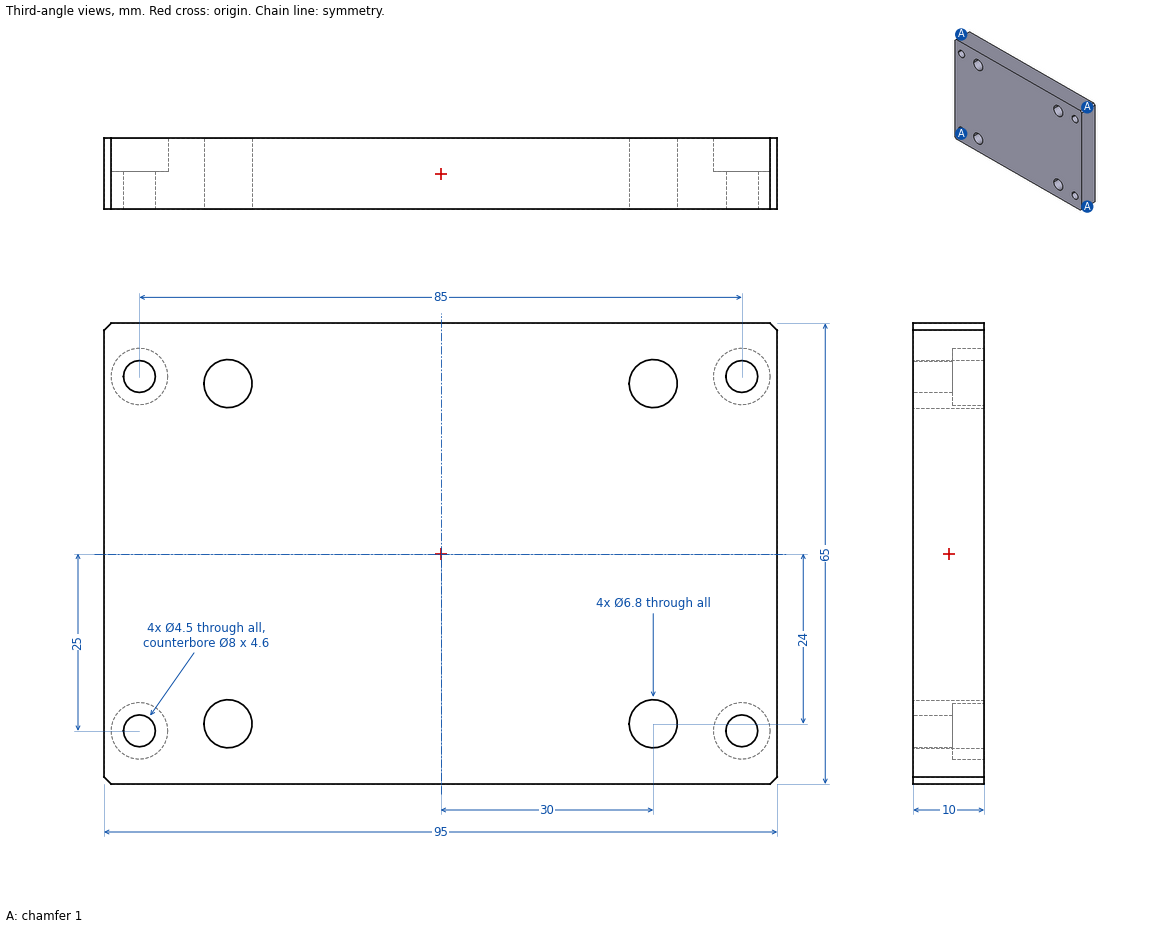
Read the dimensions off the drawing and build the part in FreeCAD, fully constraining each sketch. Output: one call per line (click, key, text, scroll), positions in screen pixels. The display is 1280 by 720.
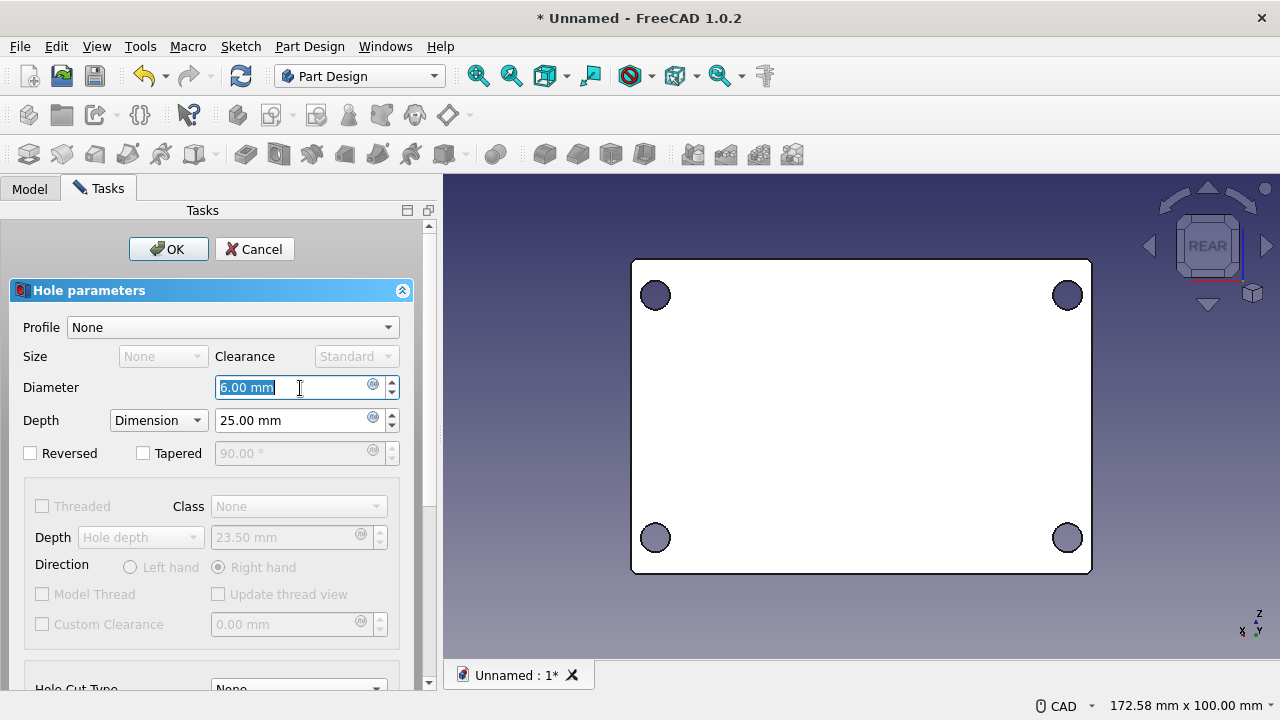
text(4.5)
key(Tab)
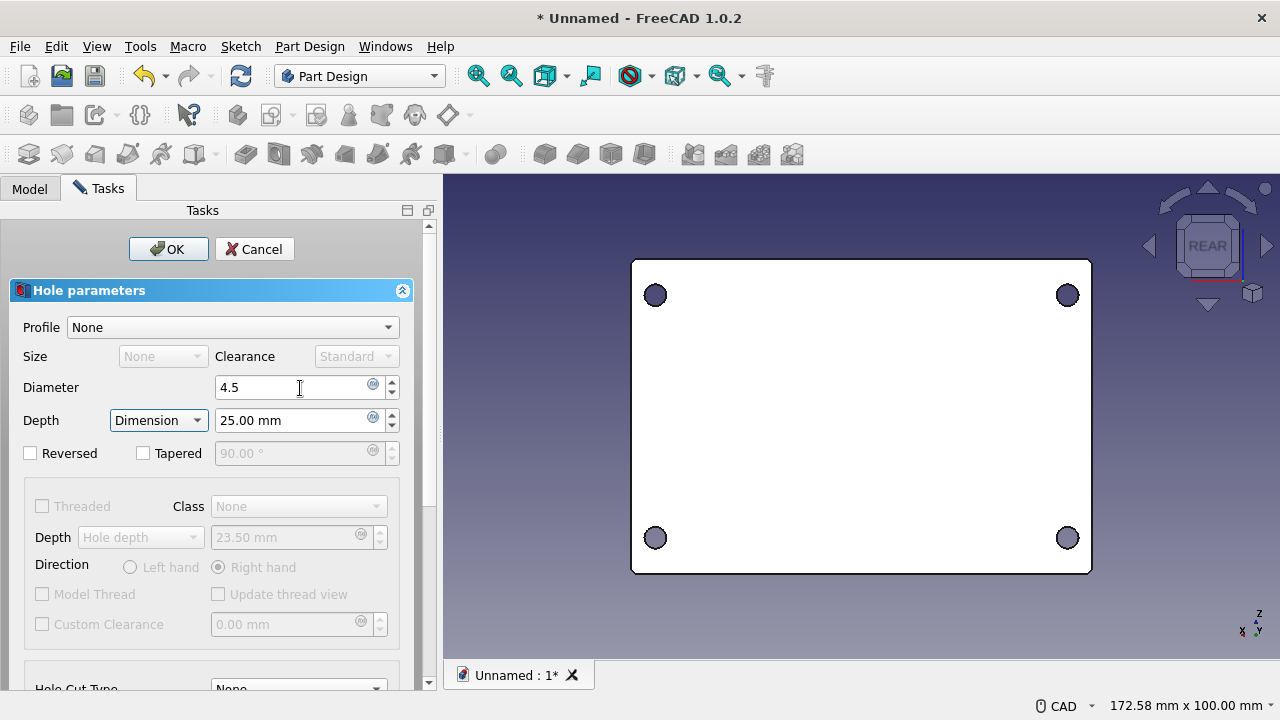
click(160, 420)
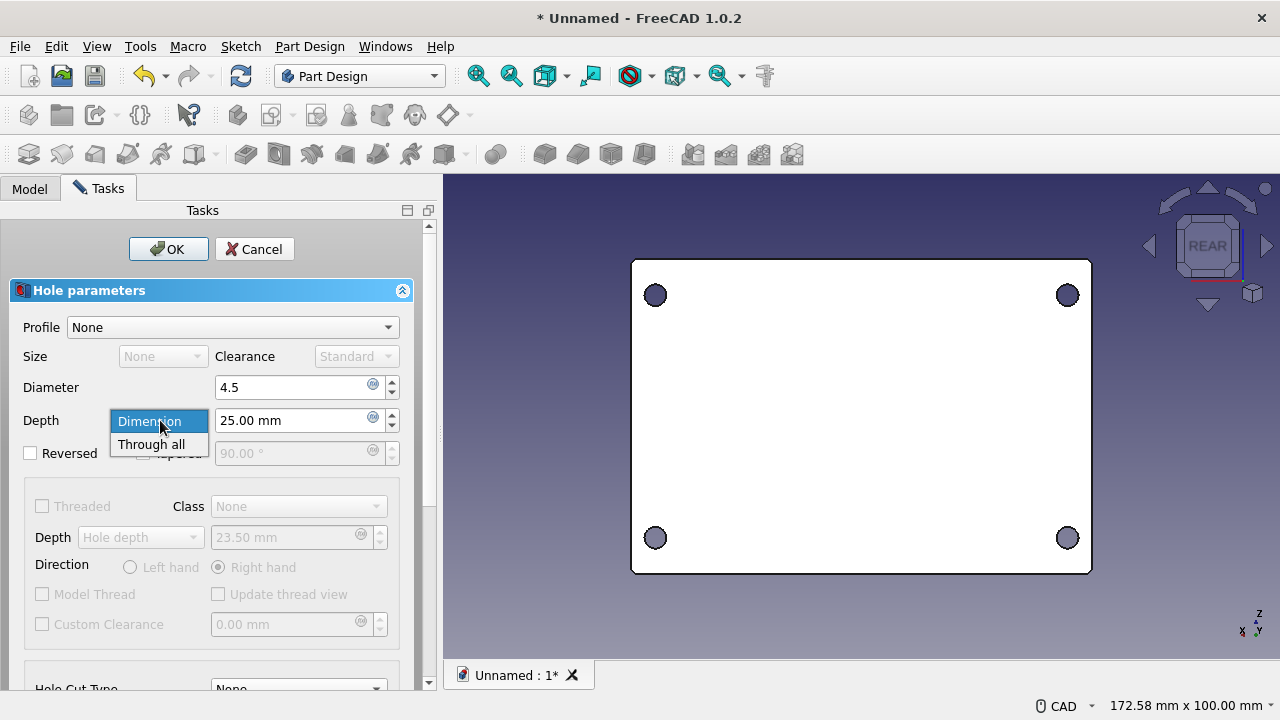
click(158, 444)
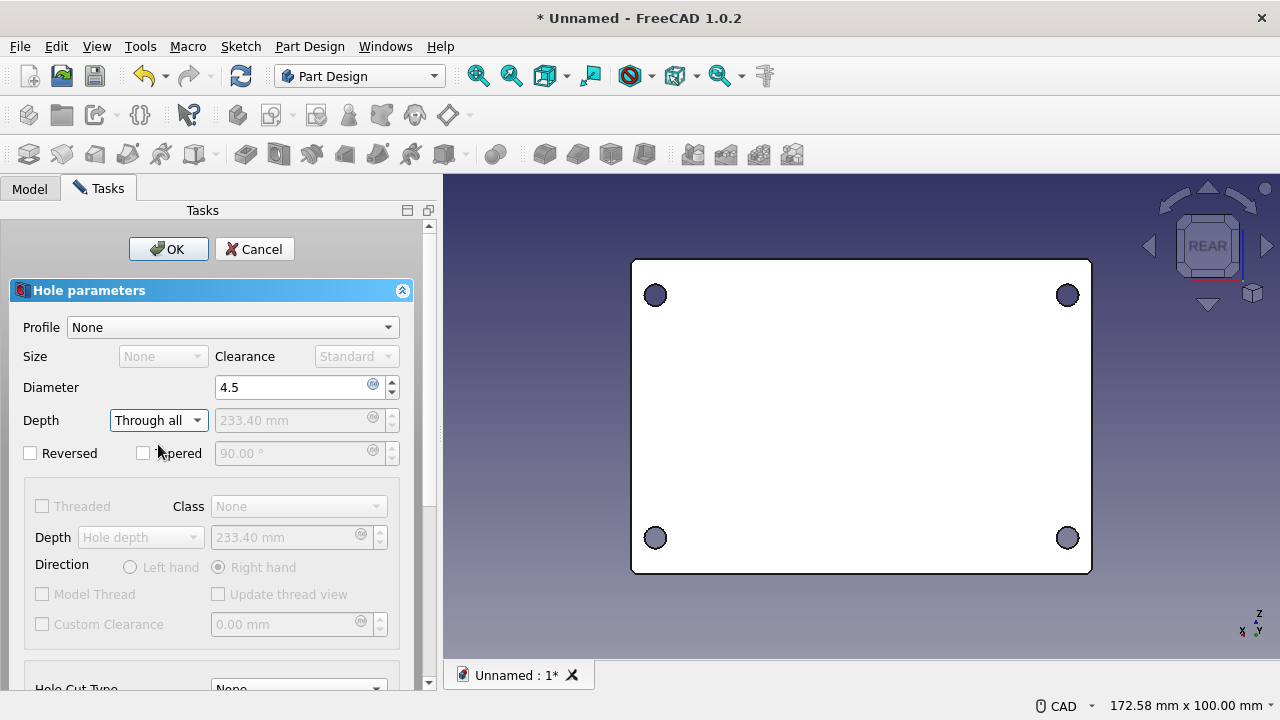
scroll(429, 455, down, 2)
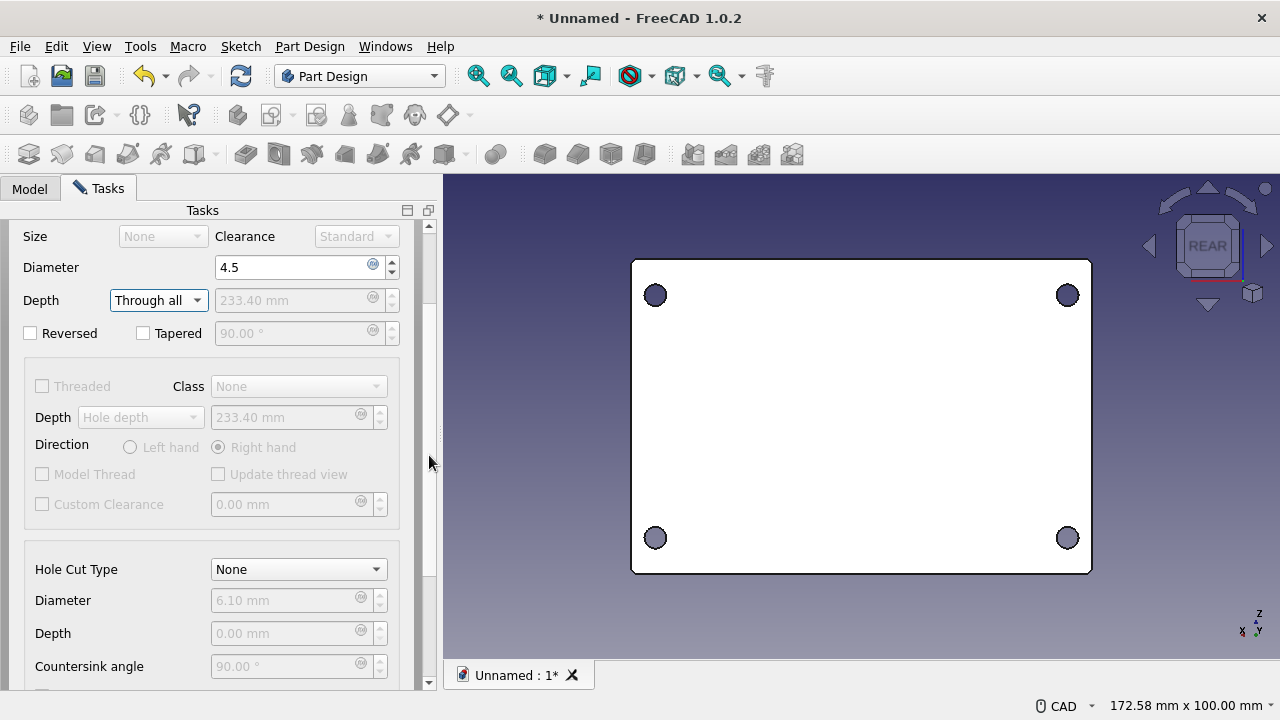
click(300, 570)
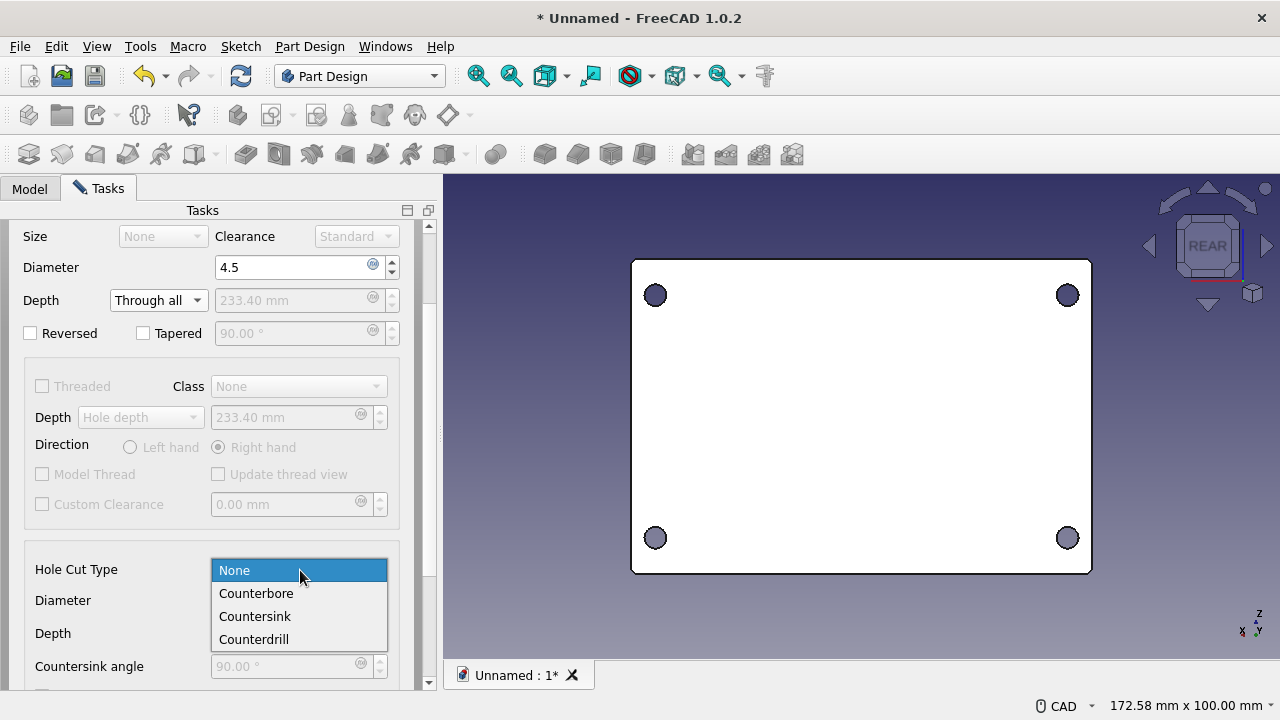
click(298, 594)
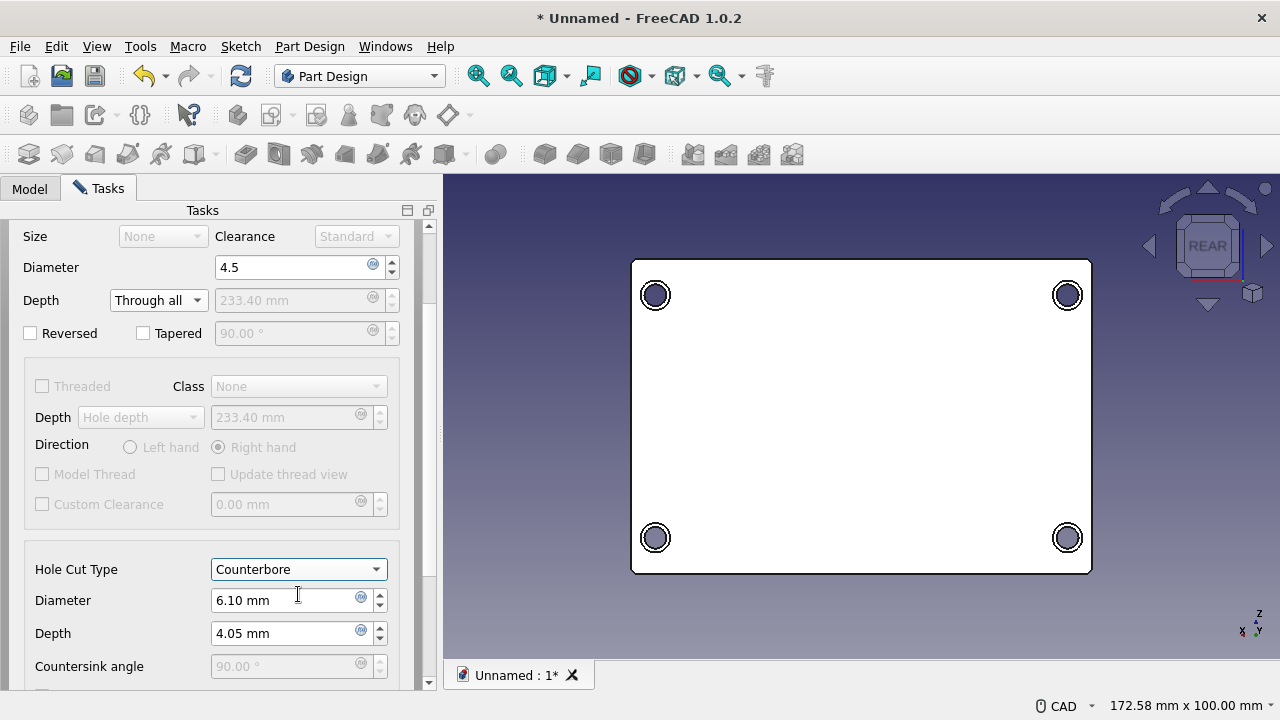
triple_click(292, 600)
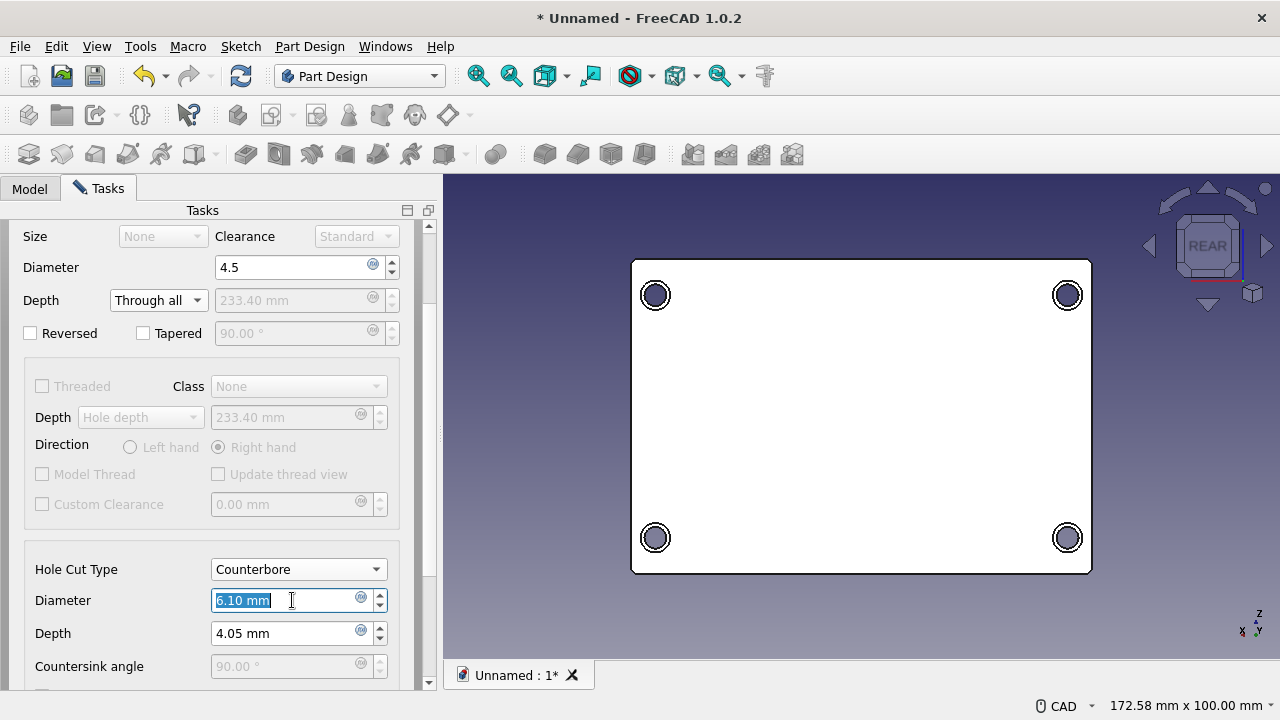
text(8)
key(Tab)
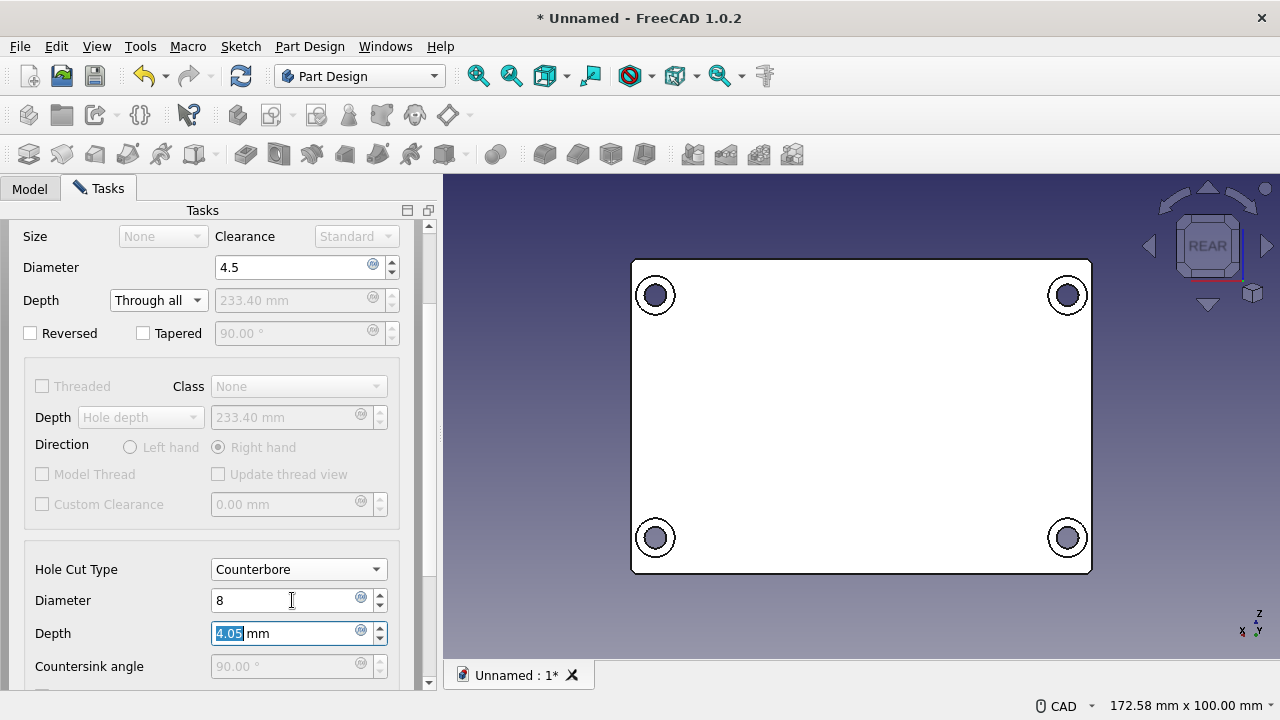
text(4.6)
key(Tab)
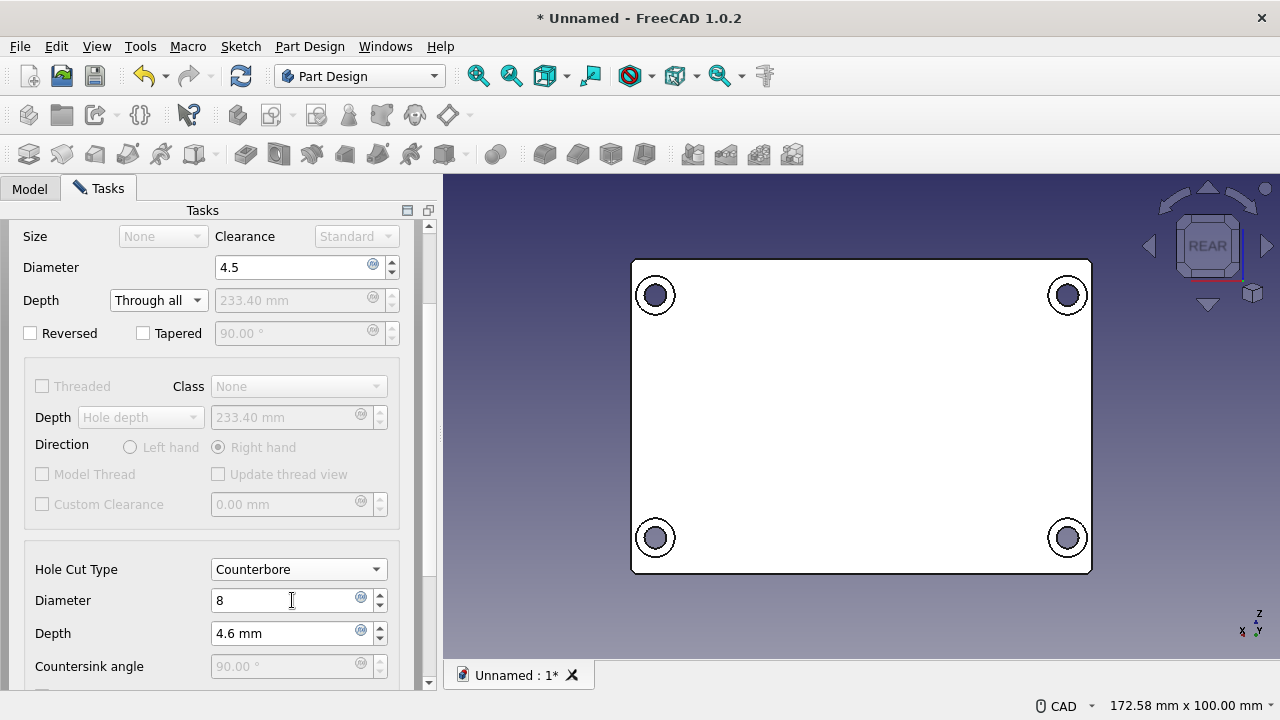
scroll(429, 455, up, 3)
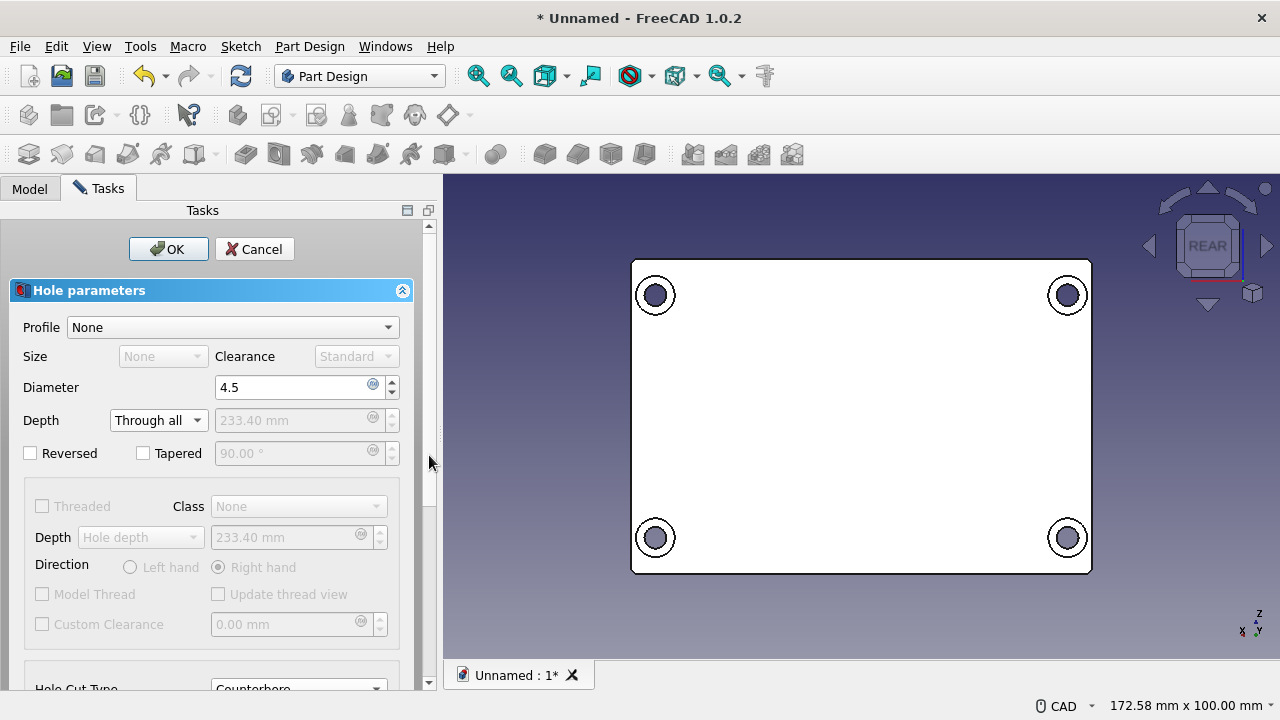
click(169, 249)